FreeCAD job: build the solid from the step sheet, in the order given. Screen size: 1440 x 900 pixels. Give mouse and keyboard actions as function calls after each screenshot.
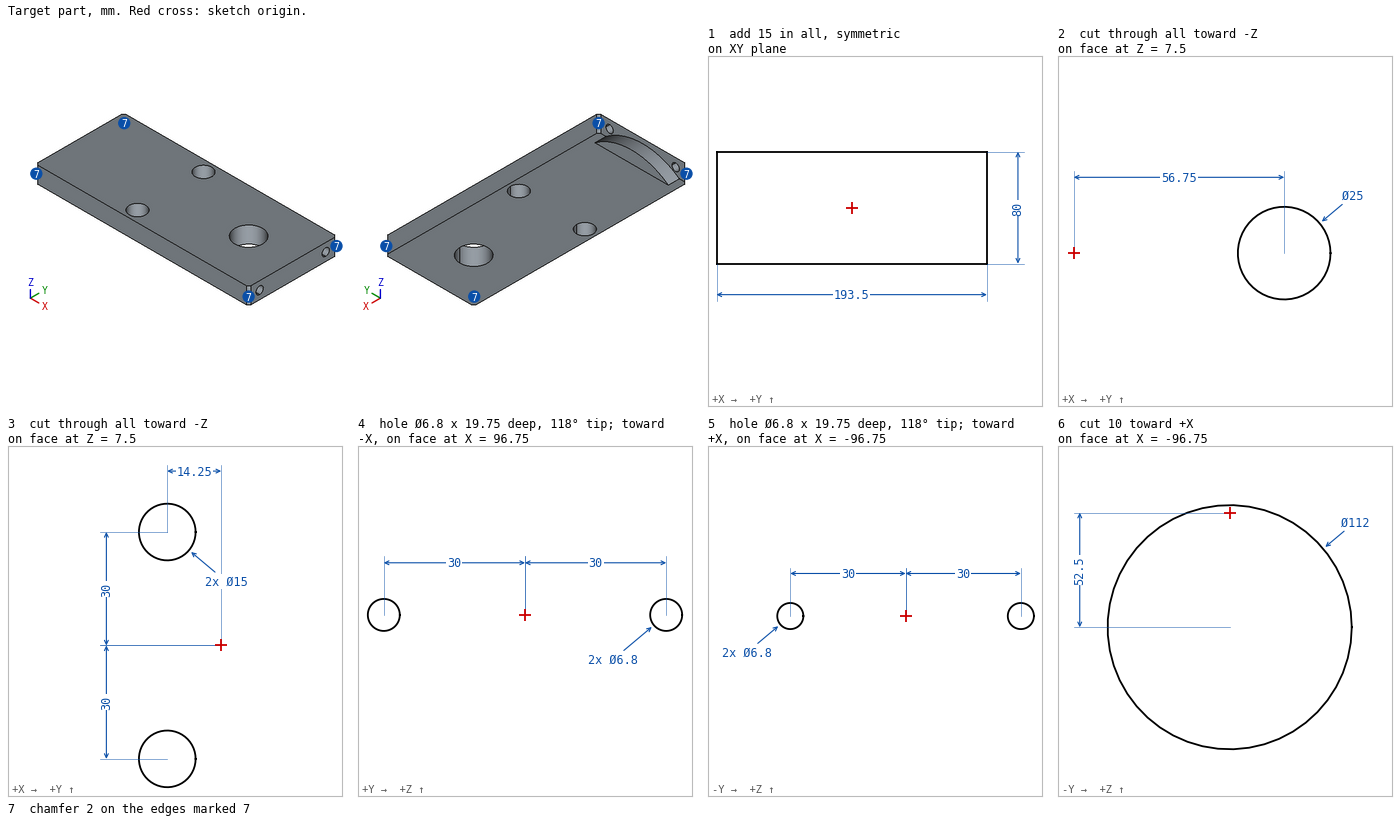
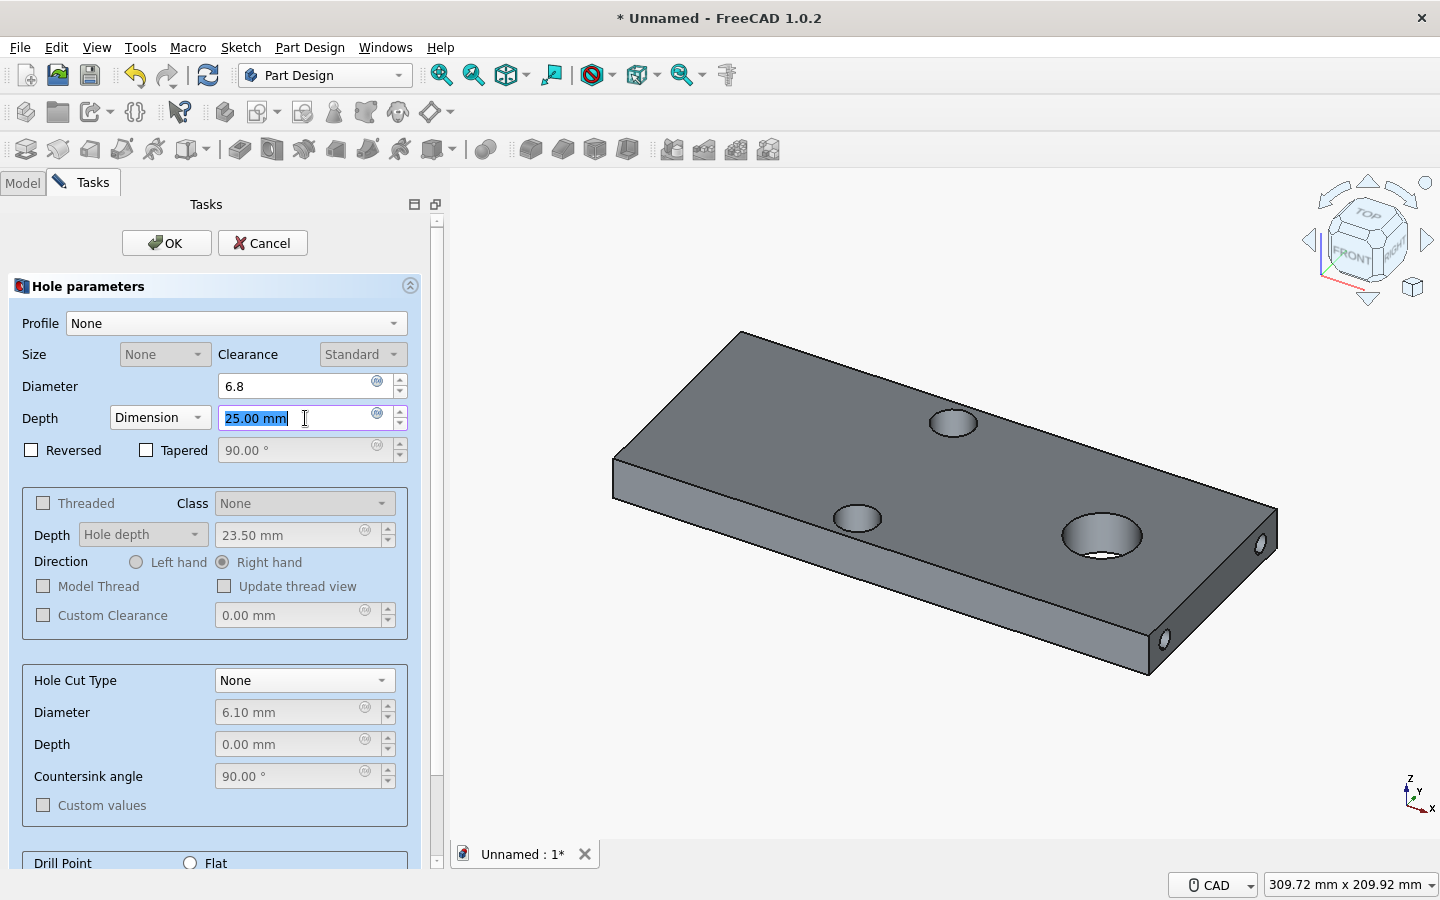
text(19.75)
key(Tab)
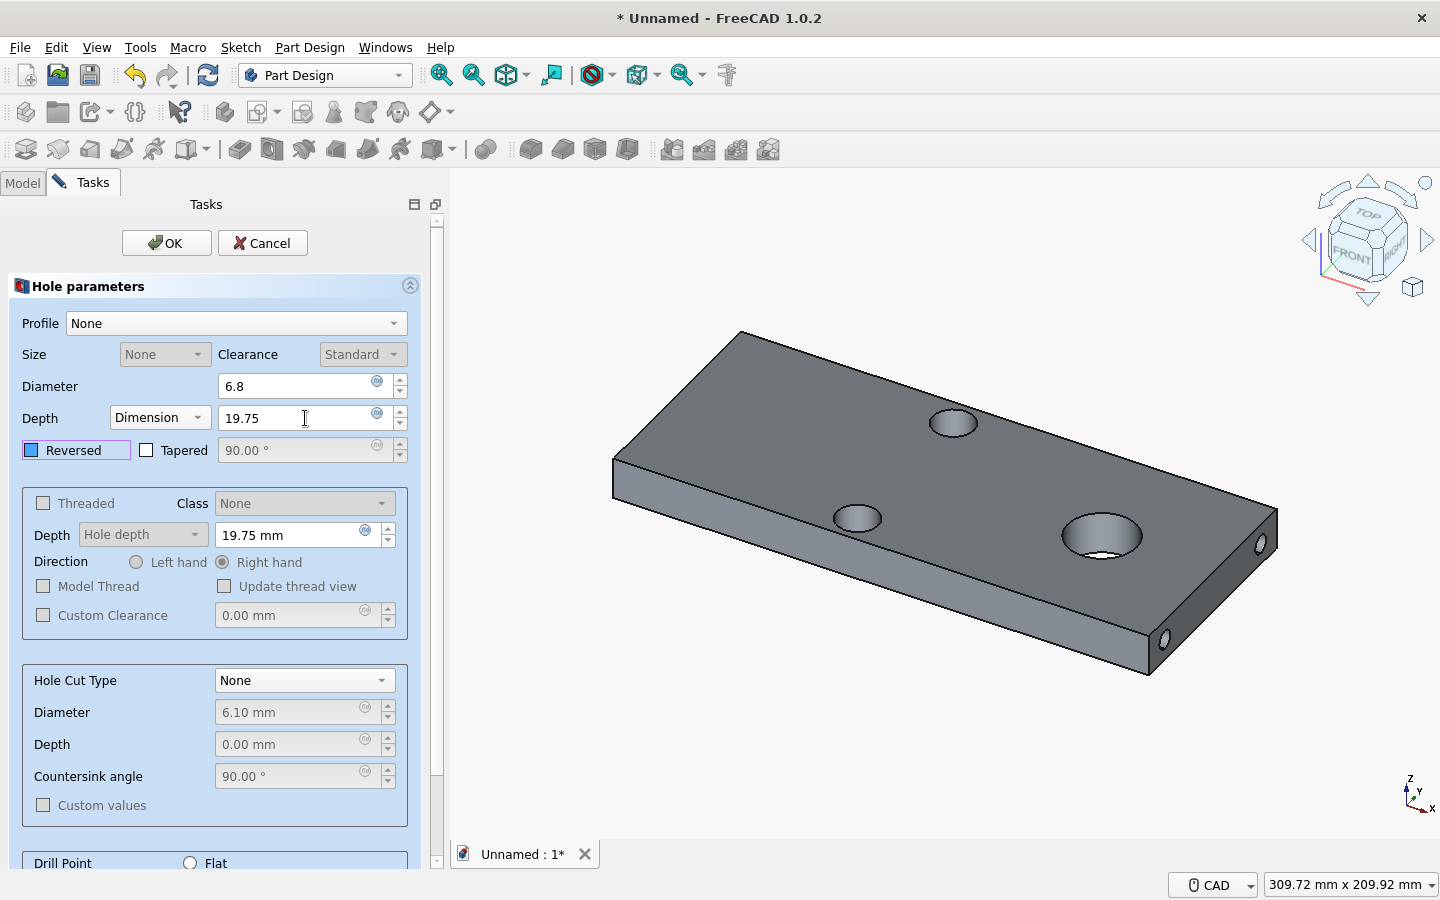
click(167, 243)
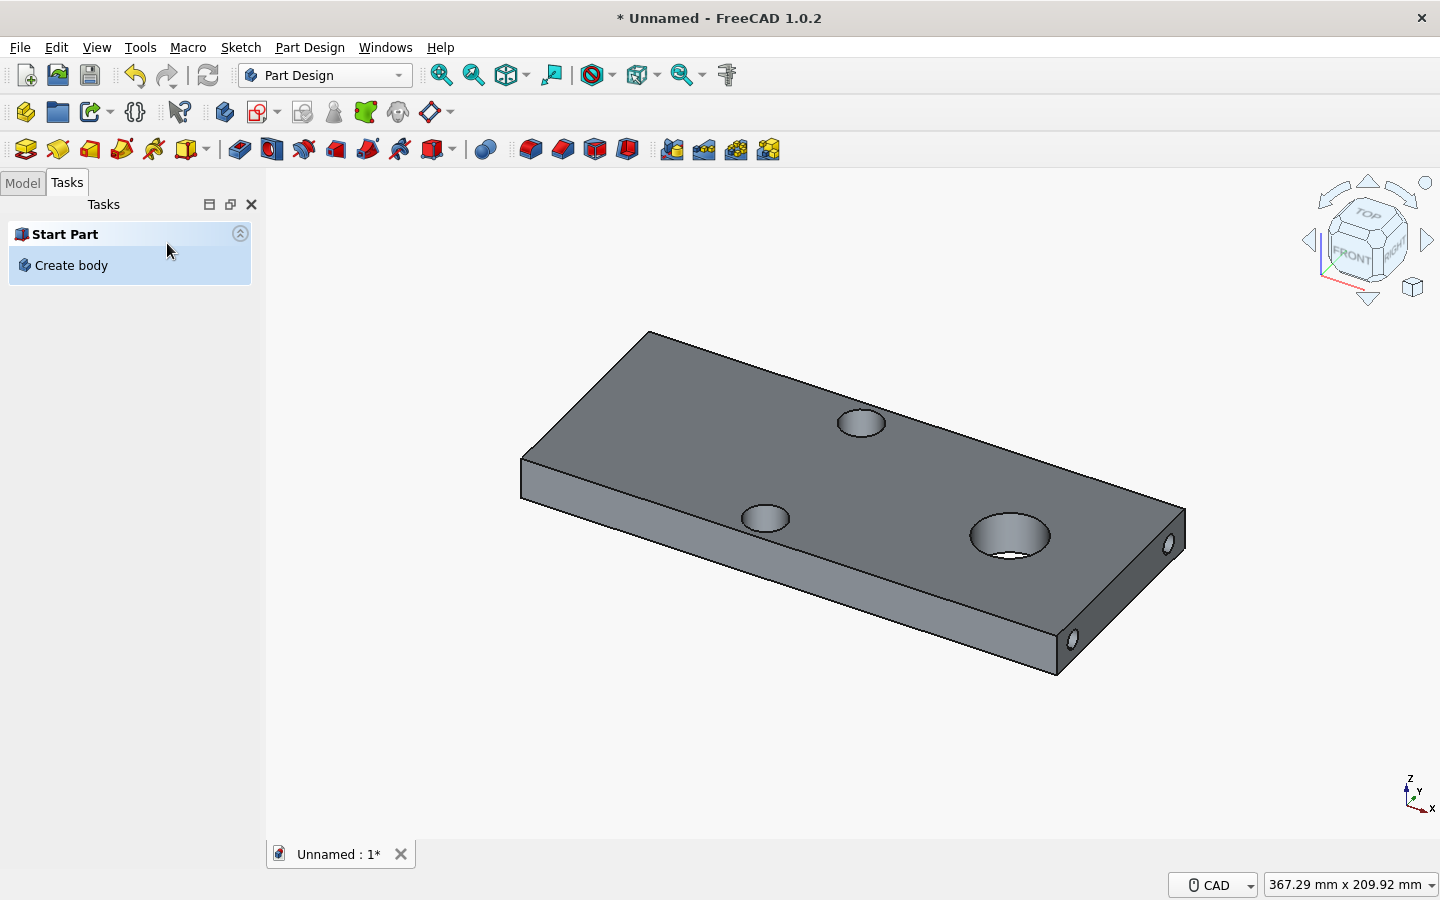
key(6)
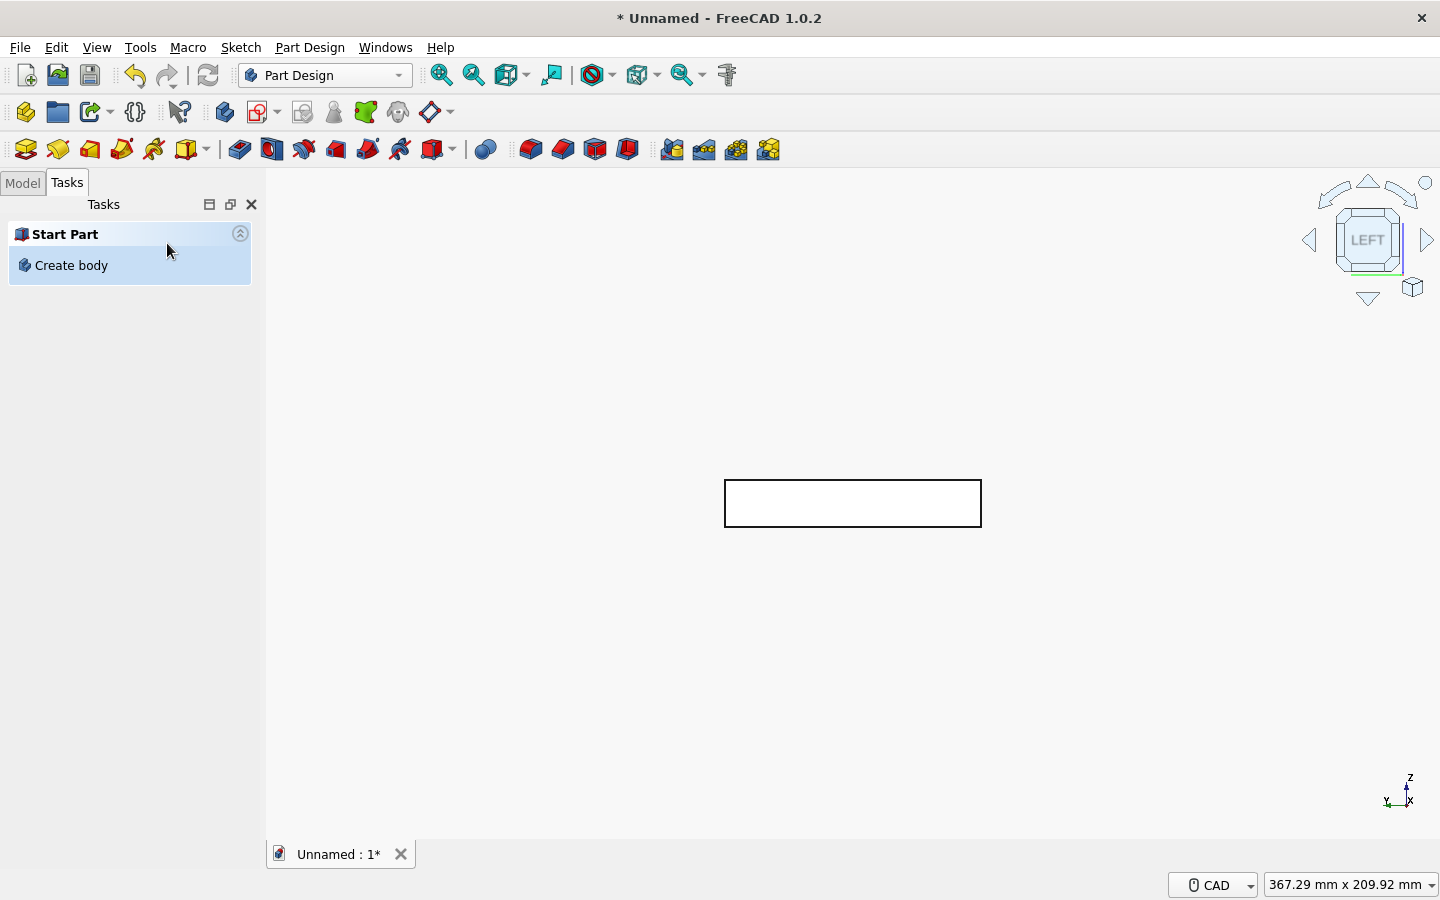
click(442, 76)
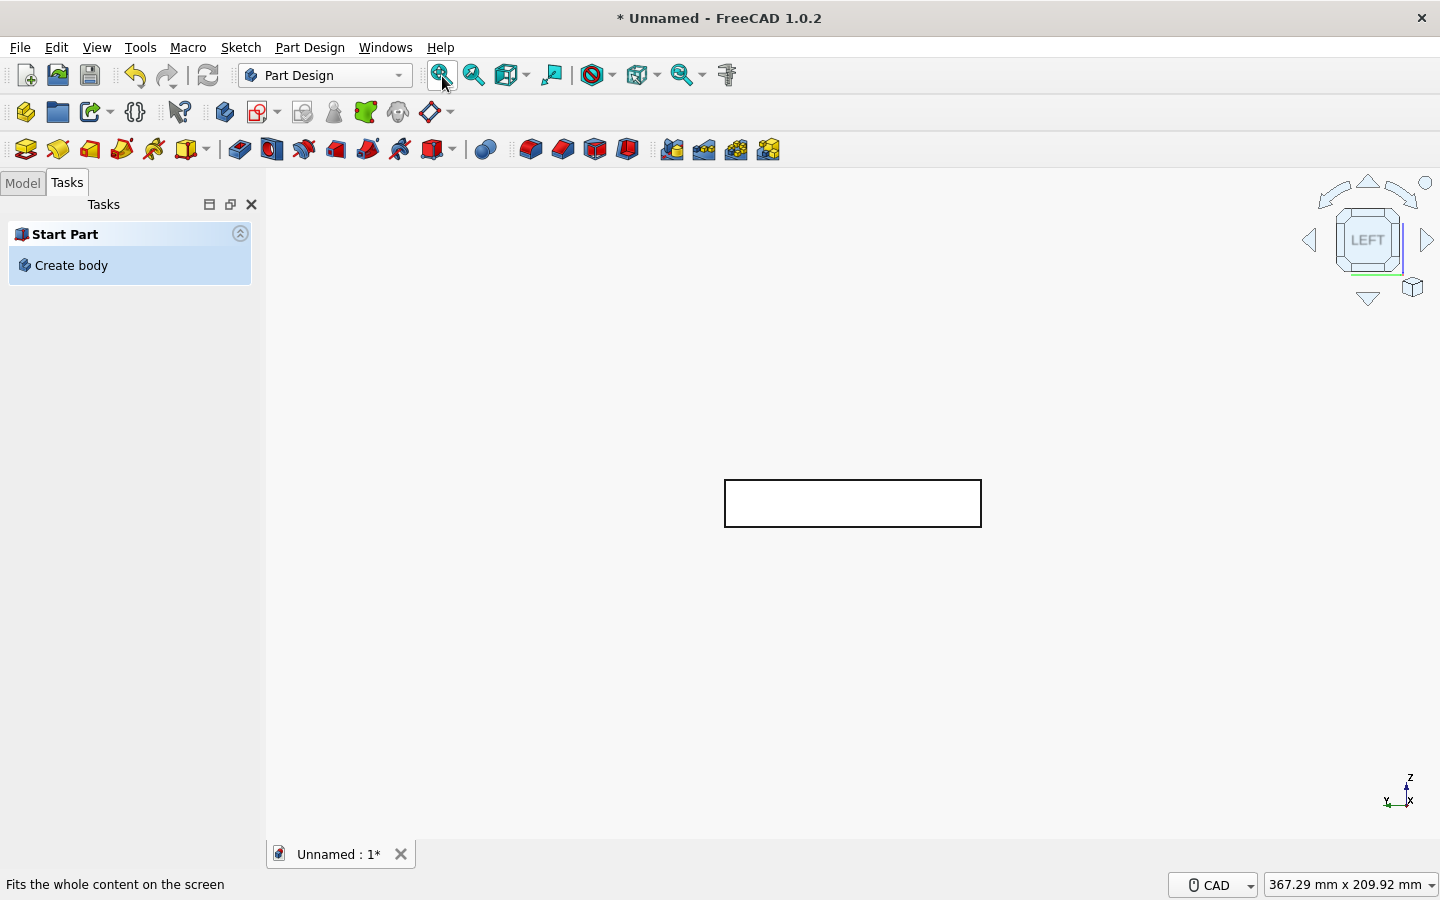
click(780, 502)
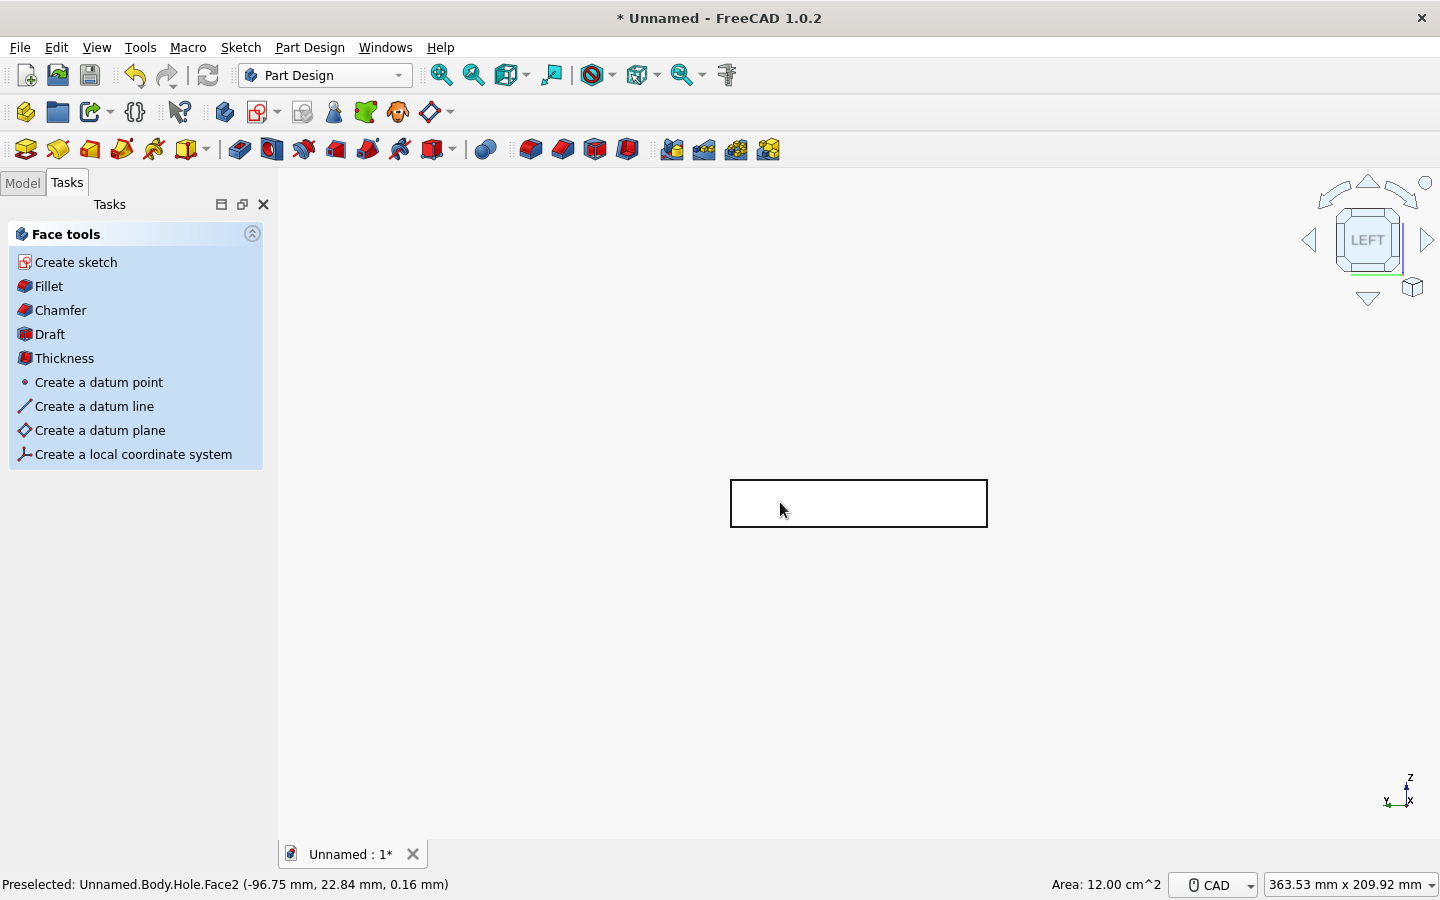
click(258, 112)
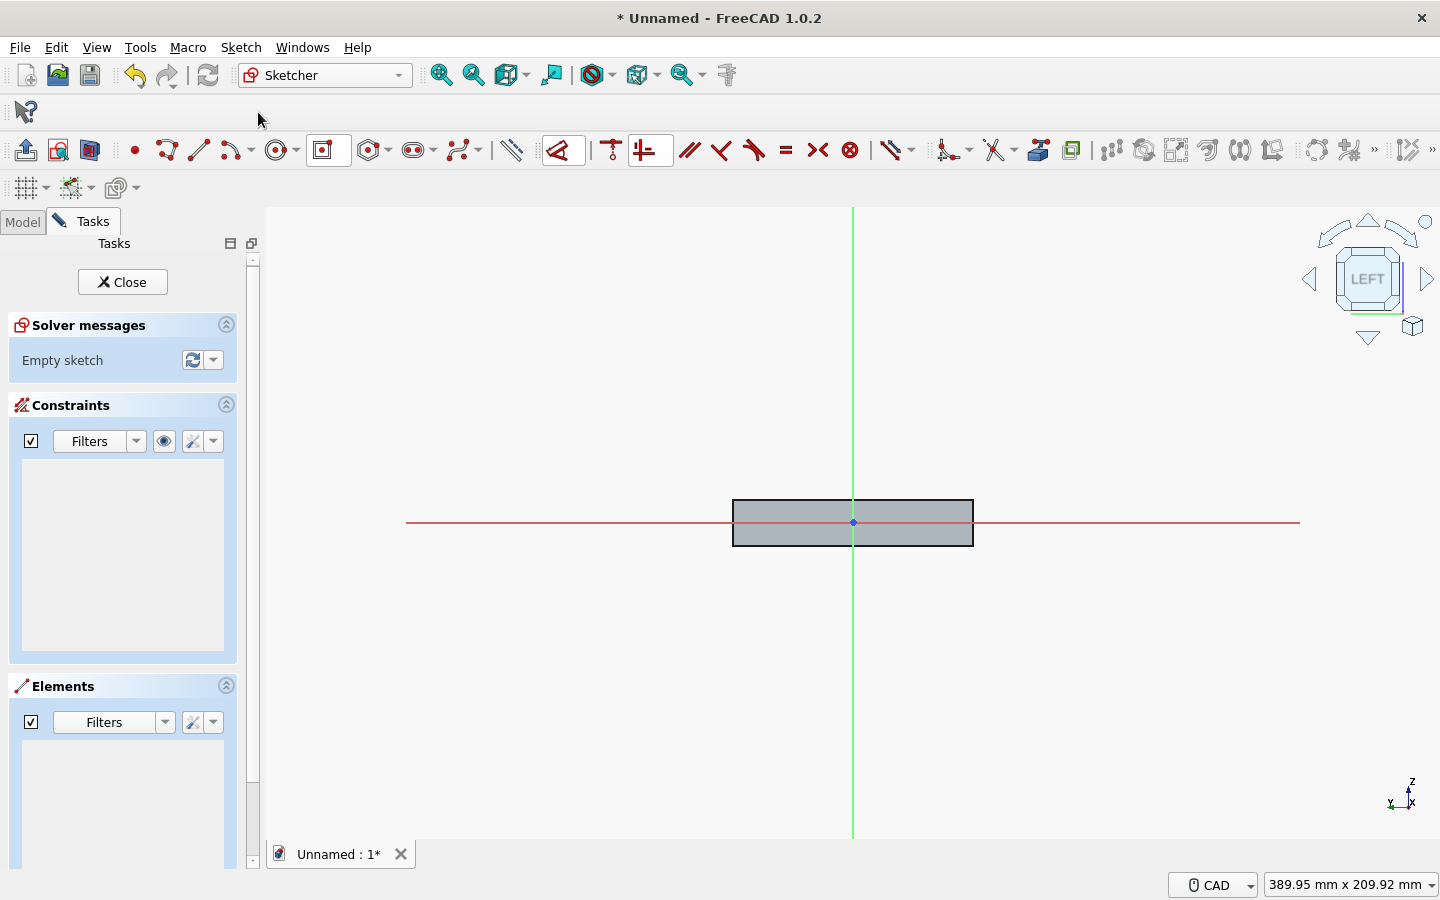
scroll(883, 523, up, 6)